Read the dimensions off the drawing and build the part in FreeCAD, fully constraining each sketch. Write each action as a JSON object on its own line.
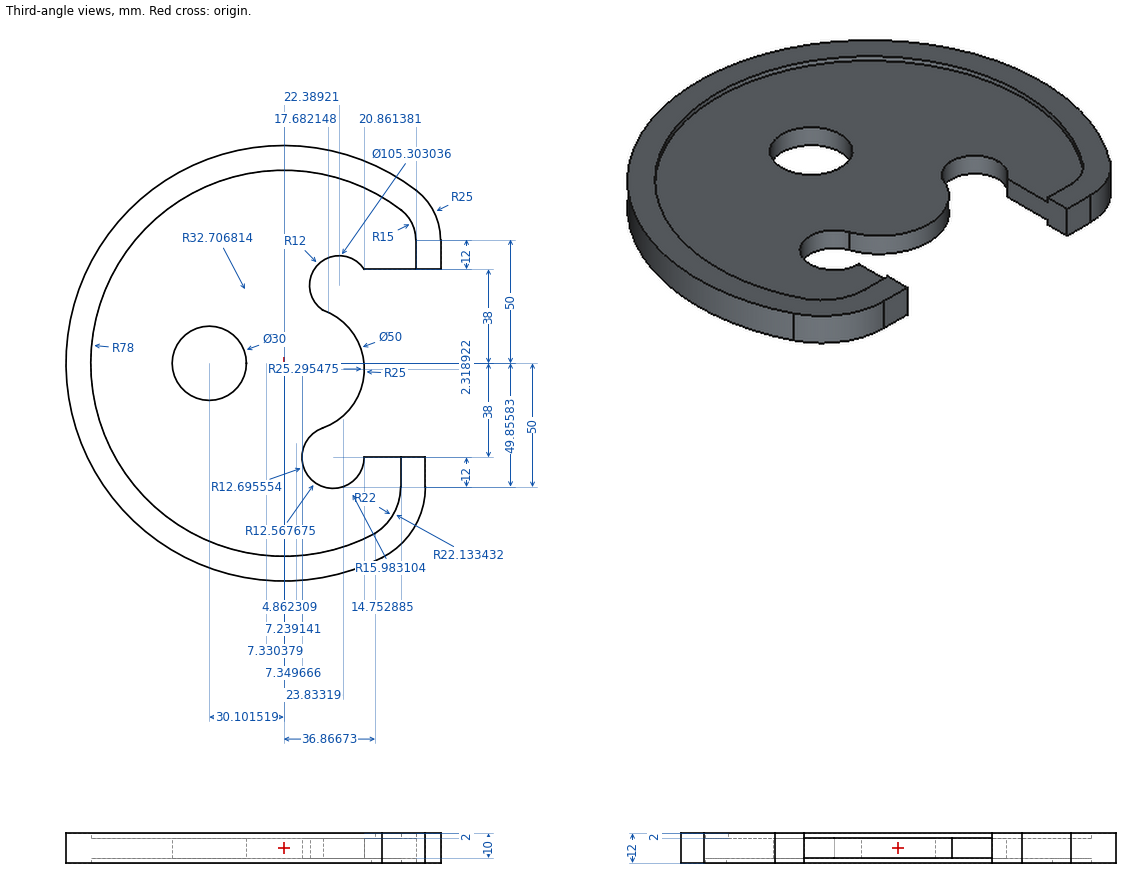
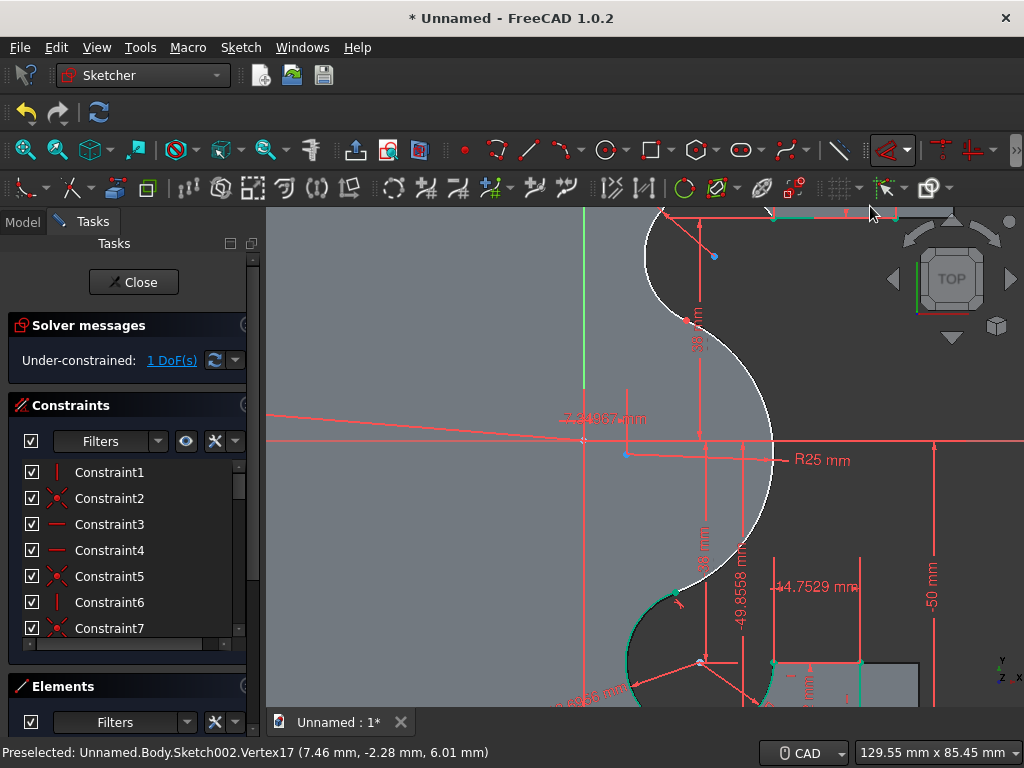
{"action": "left_click", "coordinate": [686, 321]}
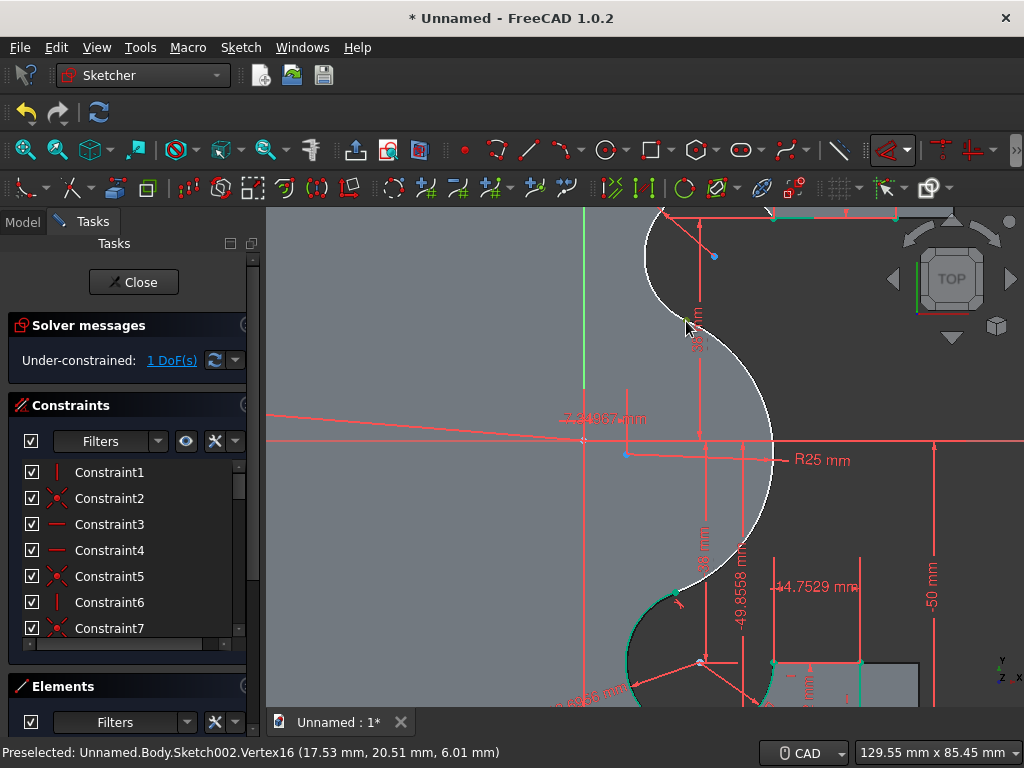
{"action": "key", "text": "l"}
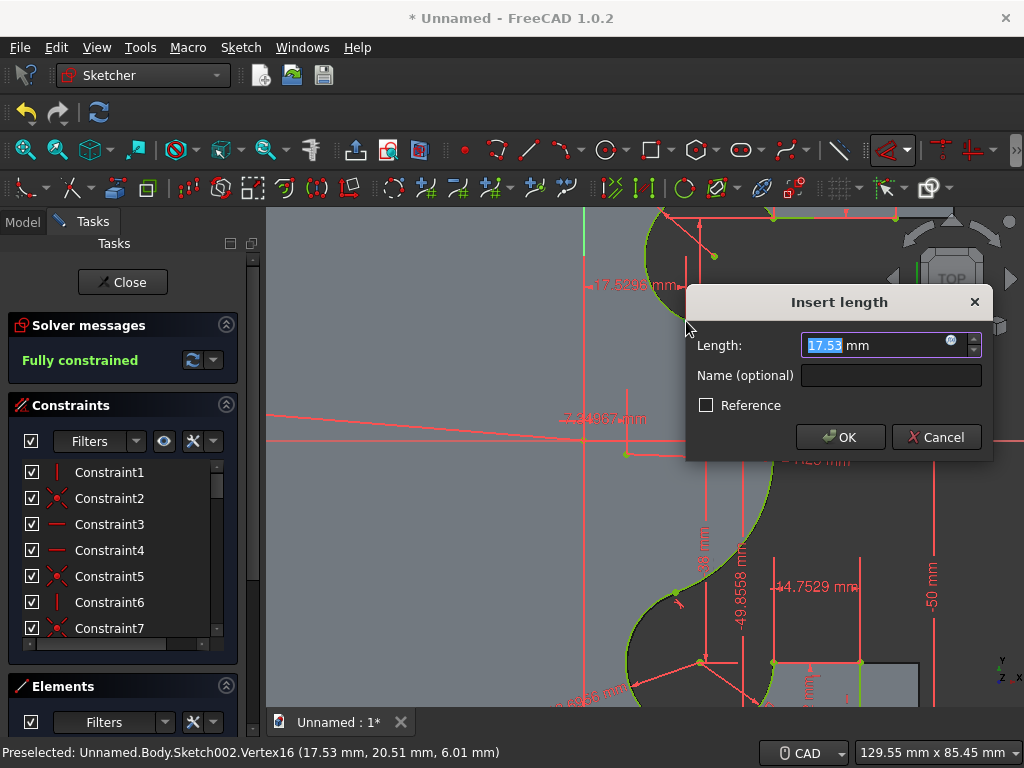
{"action": "type", "text": "17.682148"}
{"action": "key", "text": "Return"}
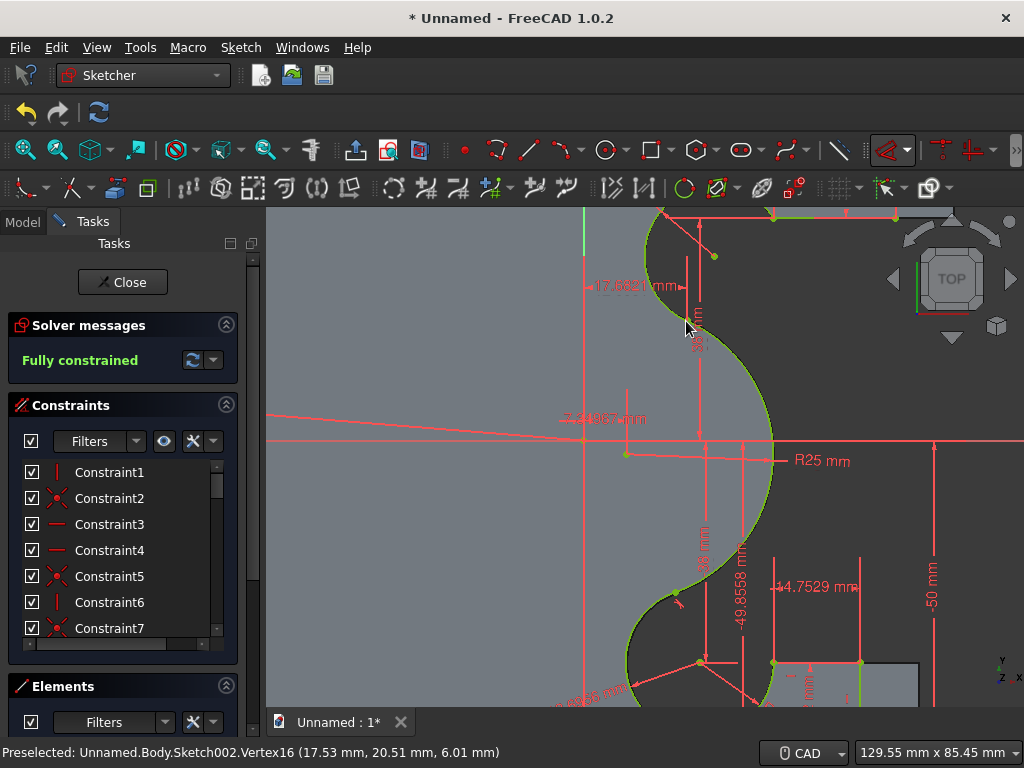
{"action": "left_click", "coordinate": [123, 282]}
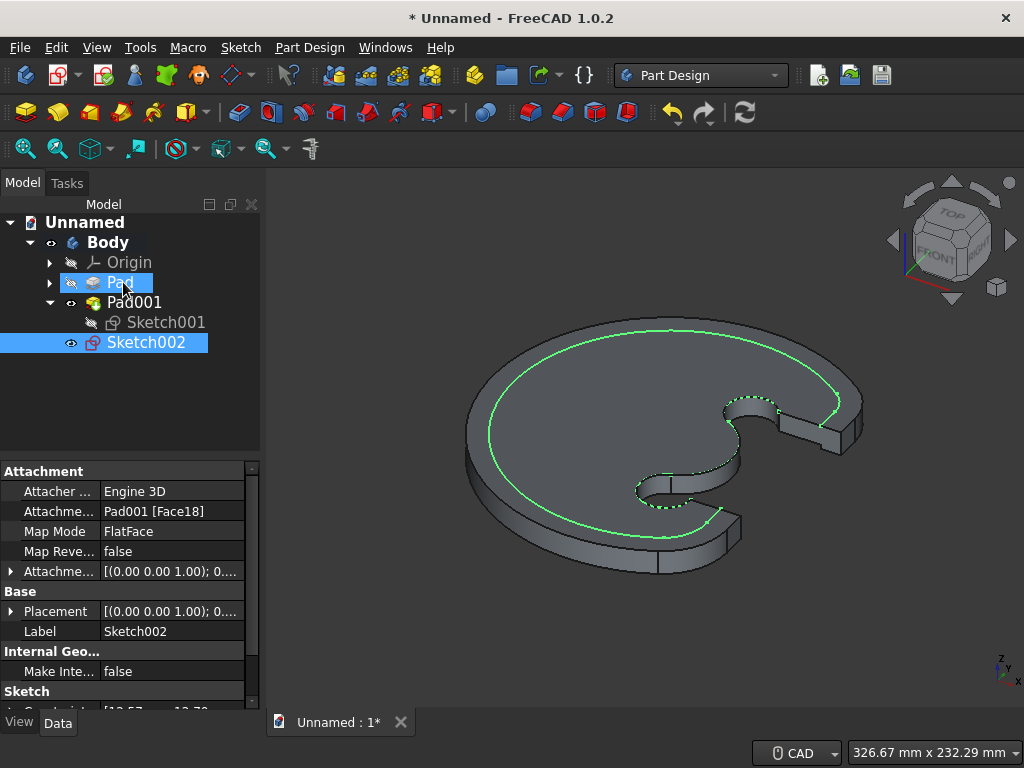
{"action": "left_click", "coordinate": [240, 112]}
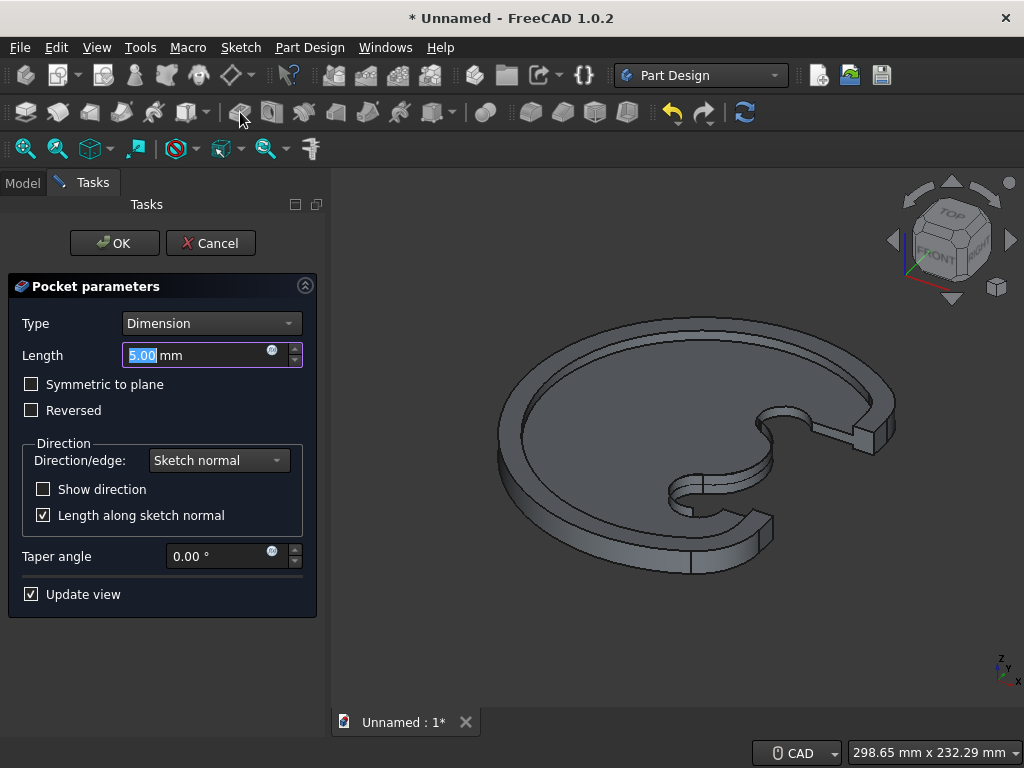
{"action": "type", "text": "2"}
{"action": "key", "text": "Tab"}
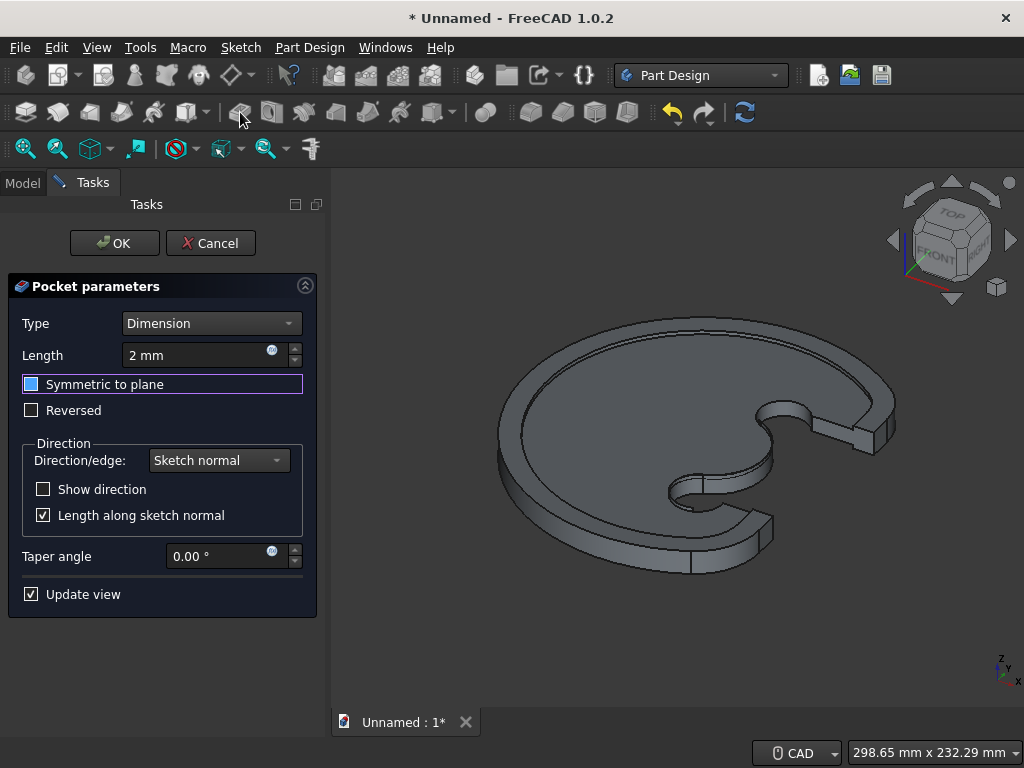
{"action": "left_click", "coordinate": [115, 243]}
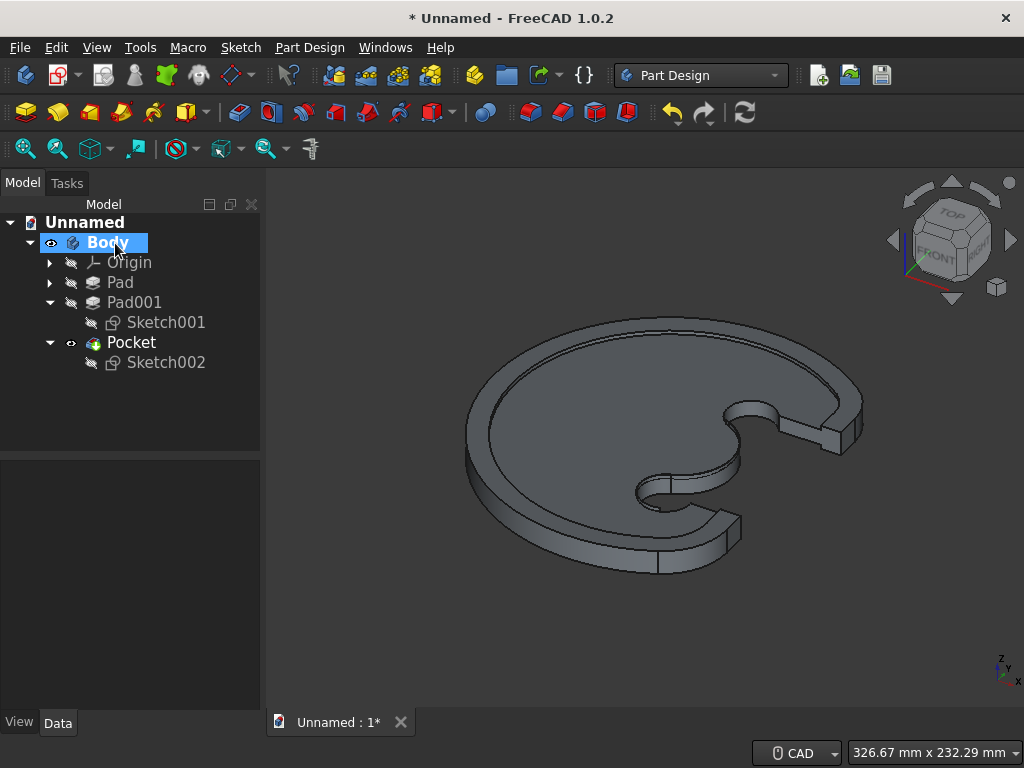
{"action": "left_click", "coordinate": [644, 541]}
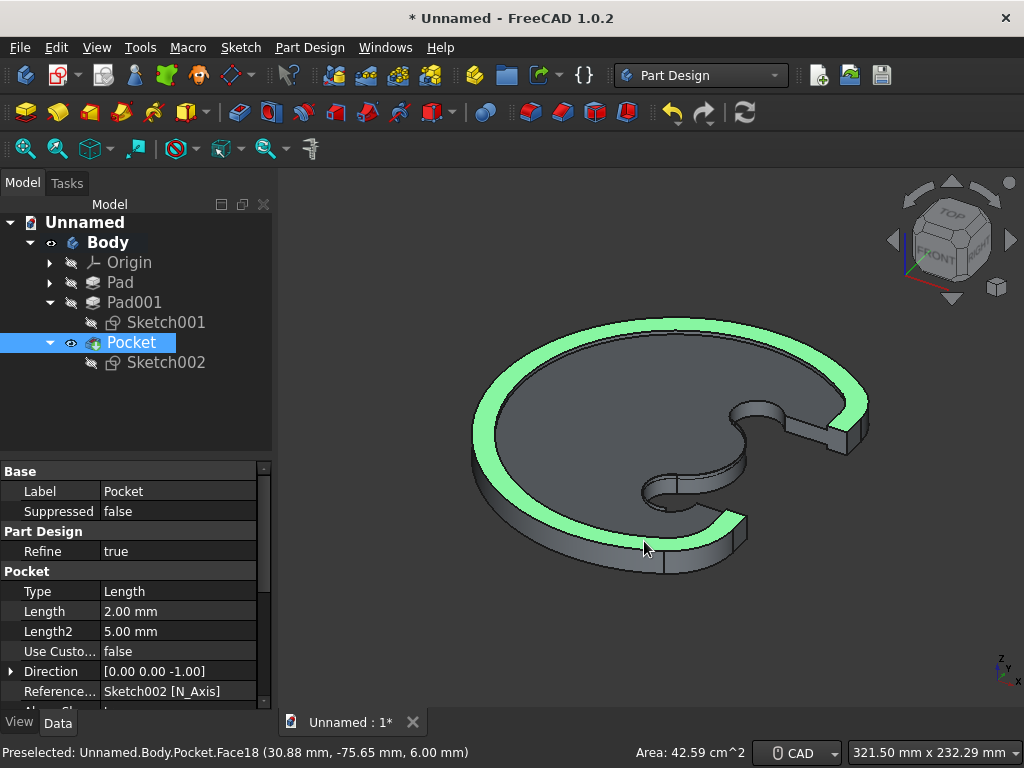
{"action": "left_click", "coordinate": [58, 76]}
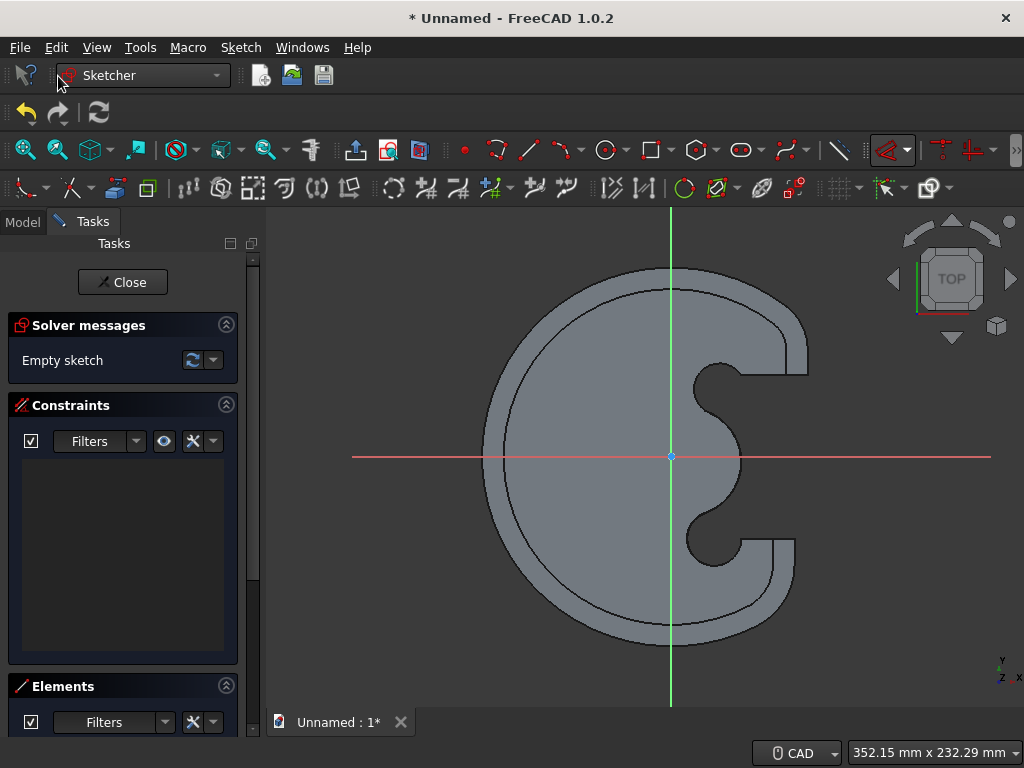
{"action": "scroll", "coordinate": [752, 465], "scroll_direction": "up", "scroll_amount": 5}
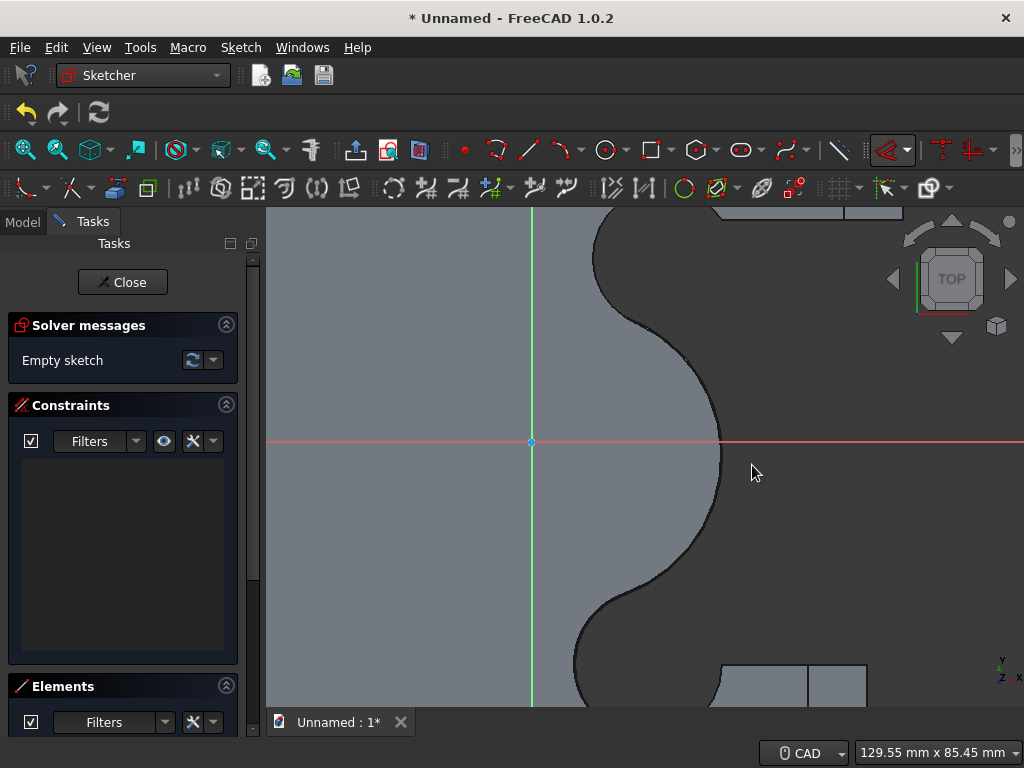
{"action": "key", "text": "g c"}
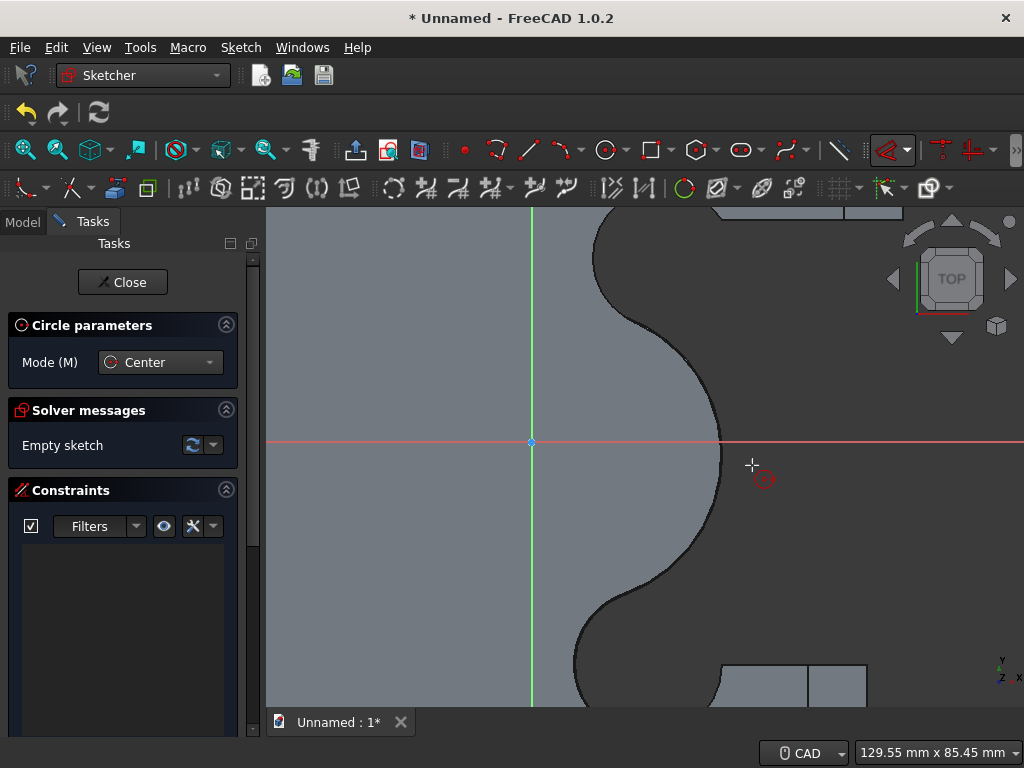
{"action": "left_click", "coordinate": [575, 456]}
{"action": "left_click", "coordinate": [678, 352]}
{"action": "key", "text": "Escape"}